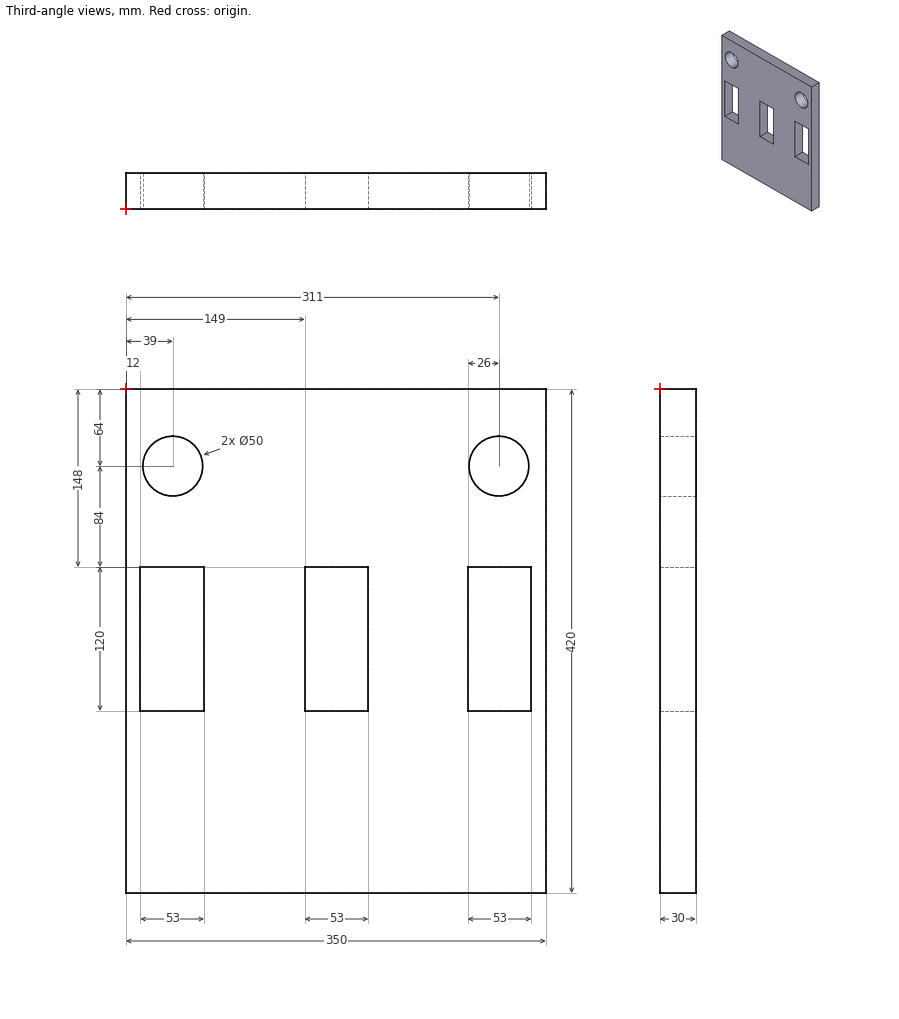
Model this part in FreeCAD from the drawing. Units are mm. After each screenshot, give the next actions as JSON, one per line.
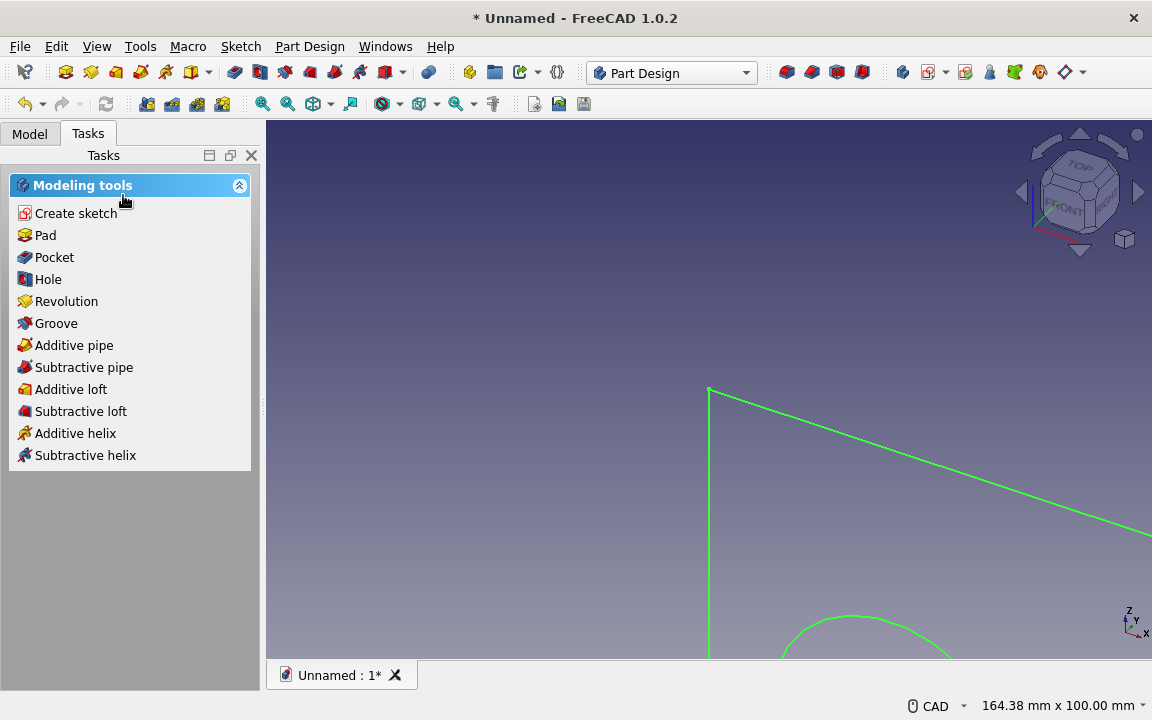
{"action": "left_click", "coordinate": [66, 72]}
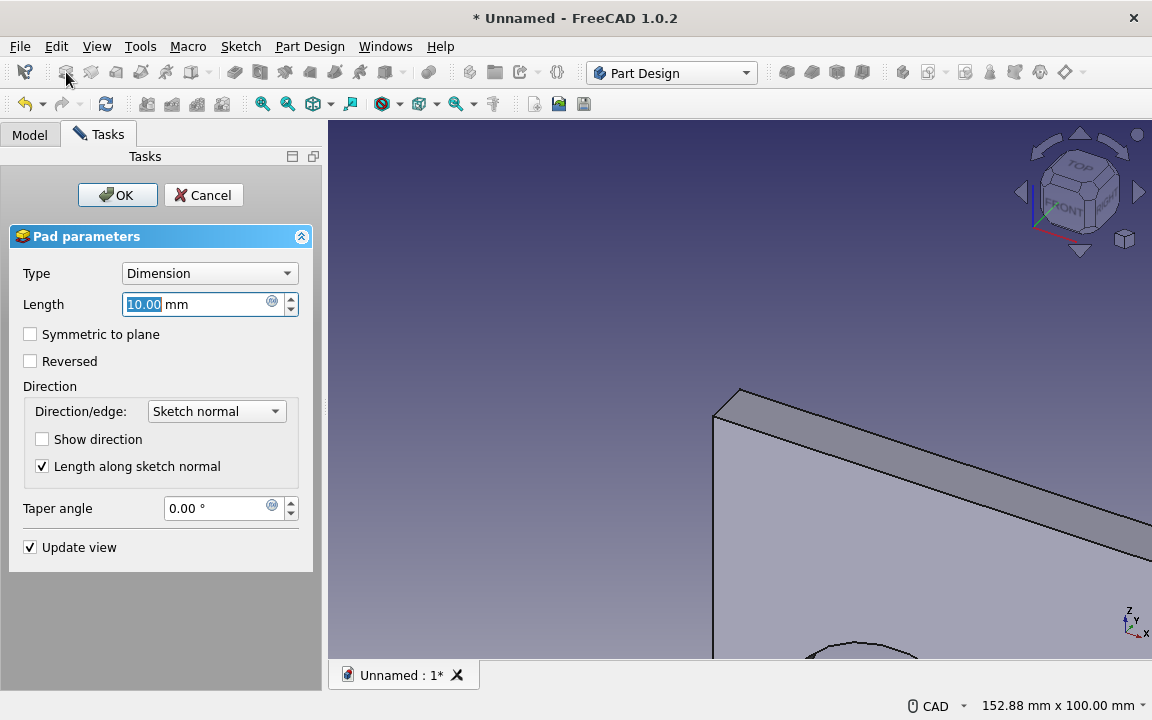
{"action": "type", "text": "30"}
{"action": "key", "text": "Tab"}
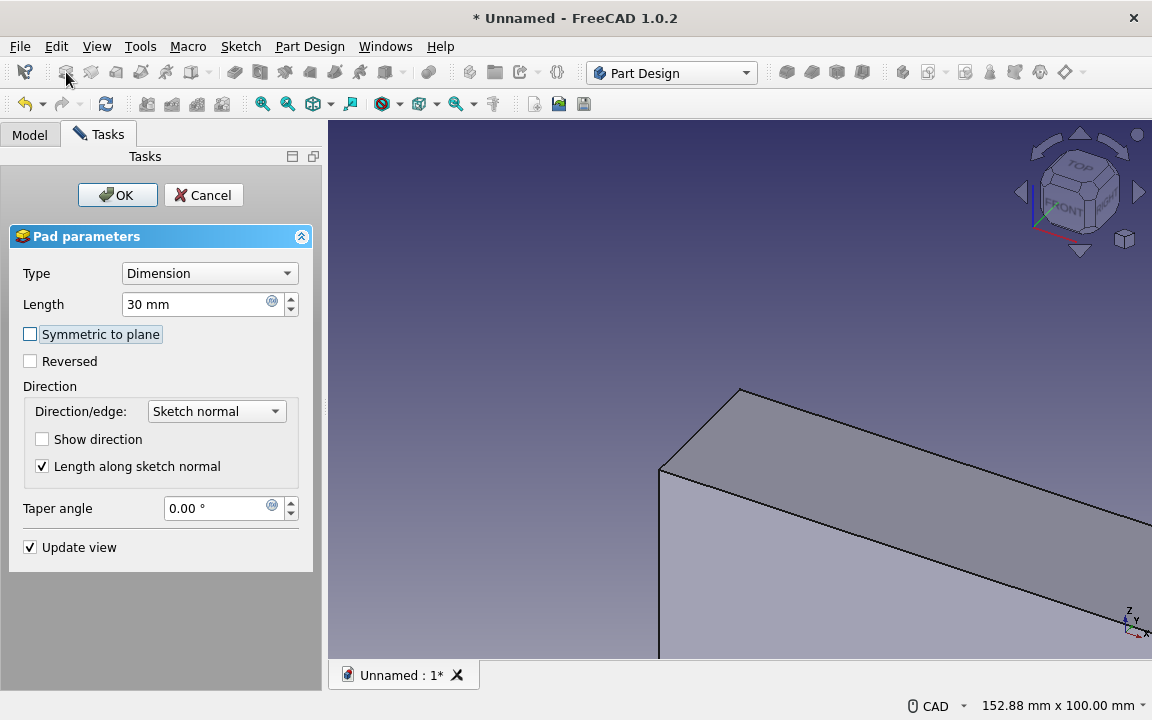
{"action": "left_click", "coordinate": [31, 361]}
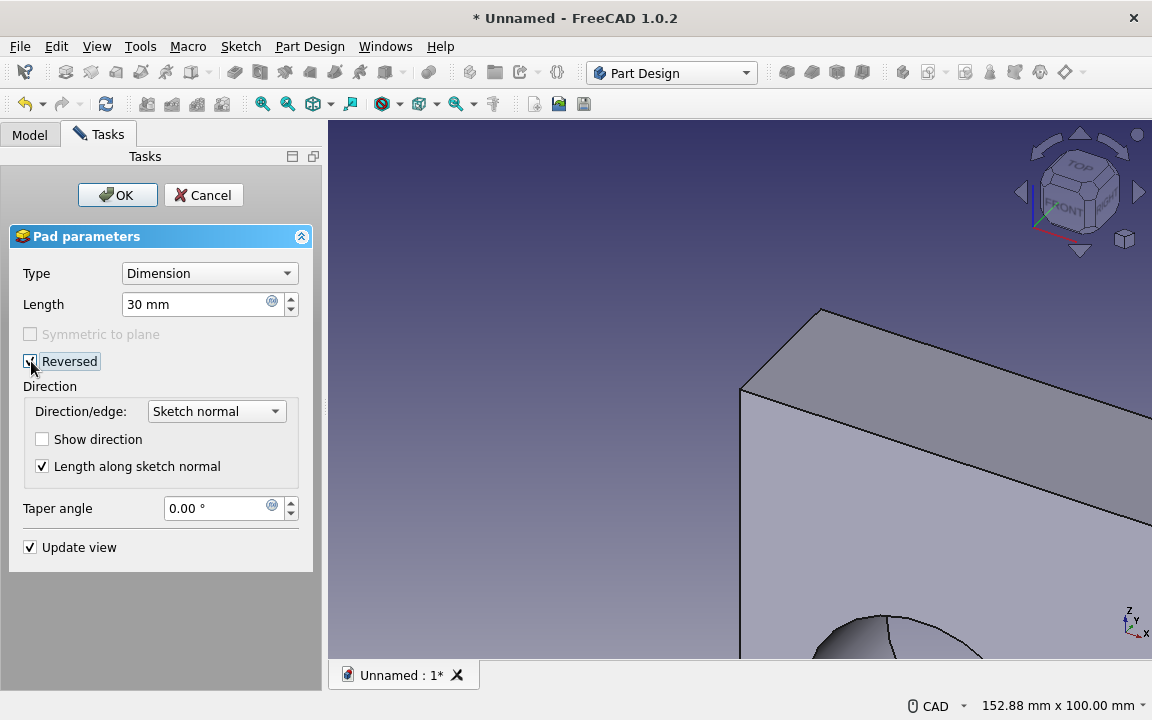
{"action": "left_click", "coordinate": [118, 195]}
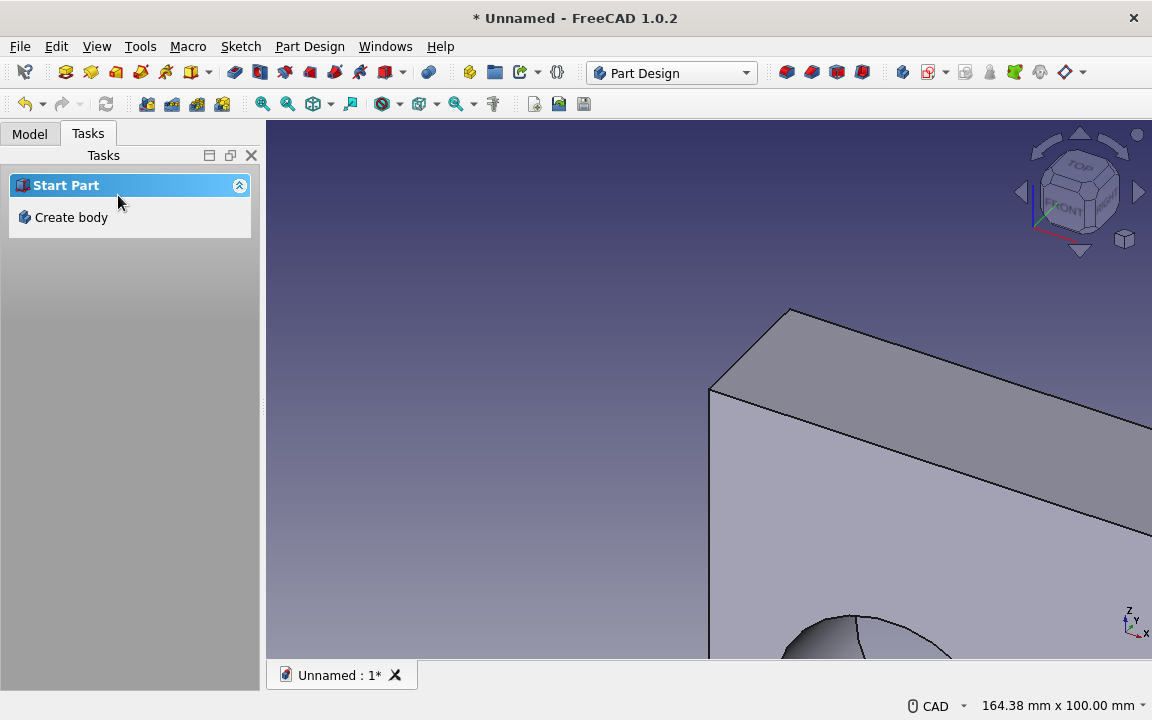
{"action": "key", "text": "0"}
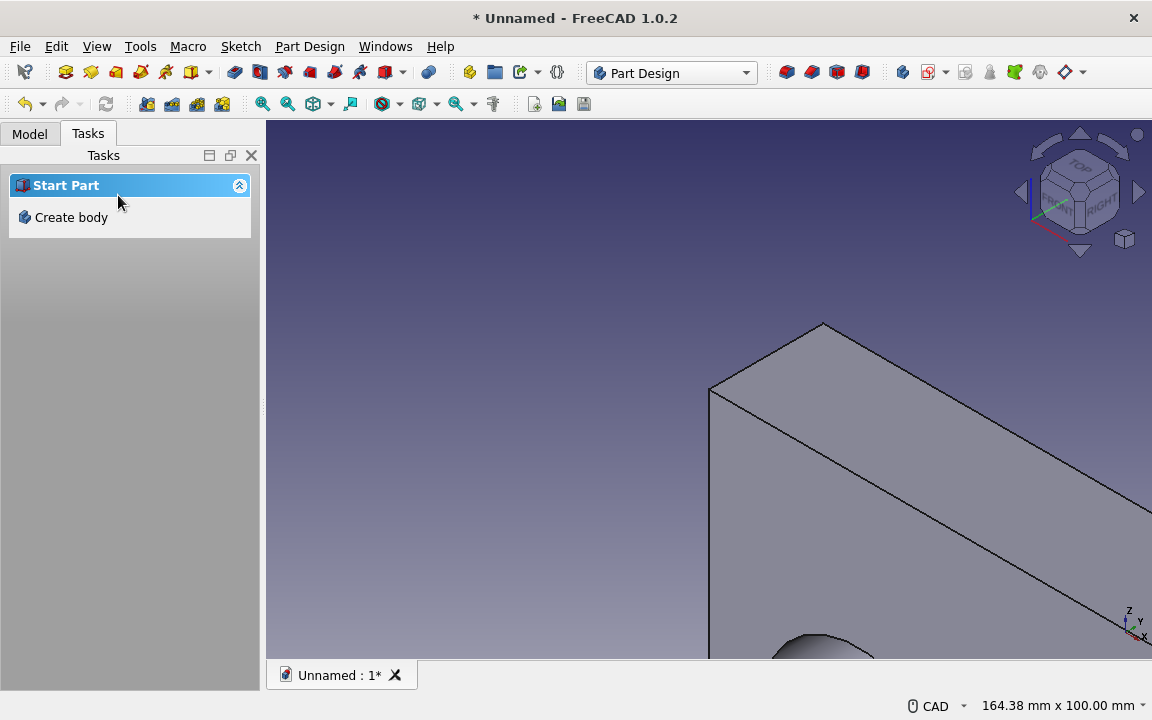
{"action": "key", "text": "v f"}